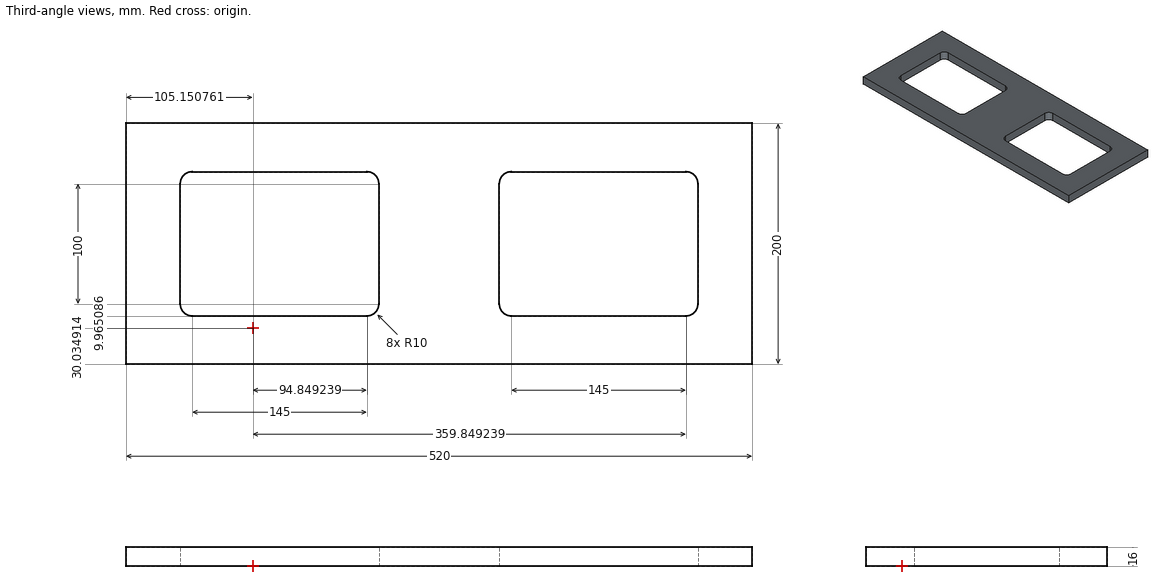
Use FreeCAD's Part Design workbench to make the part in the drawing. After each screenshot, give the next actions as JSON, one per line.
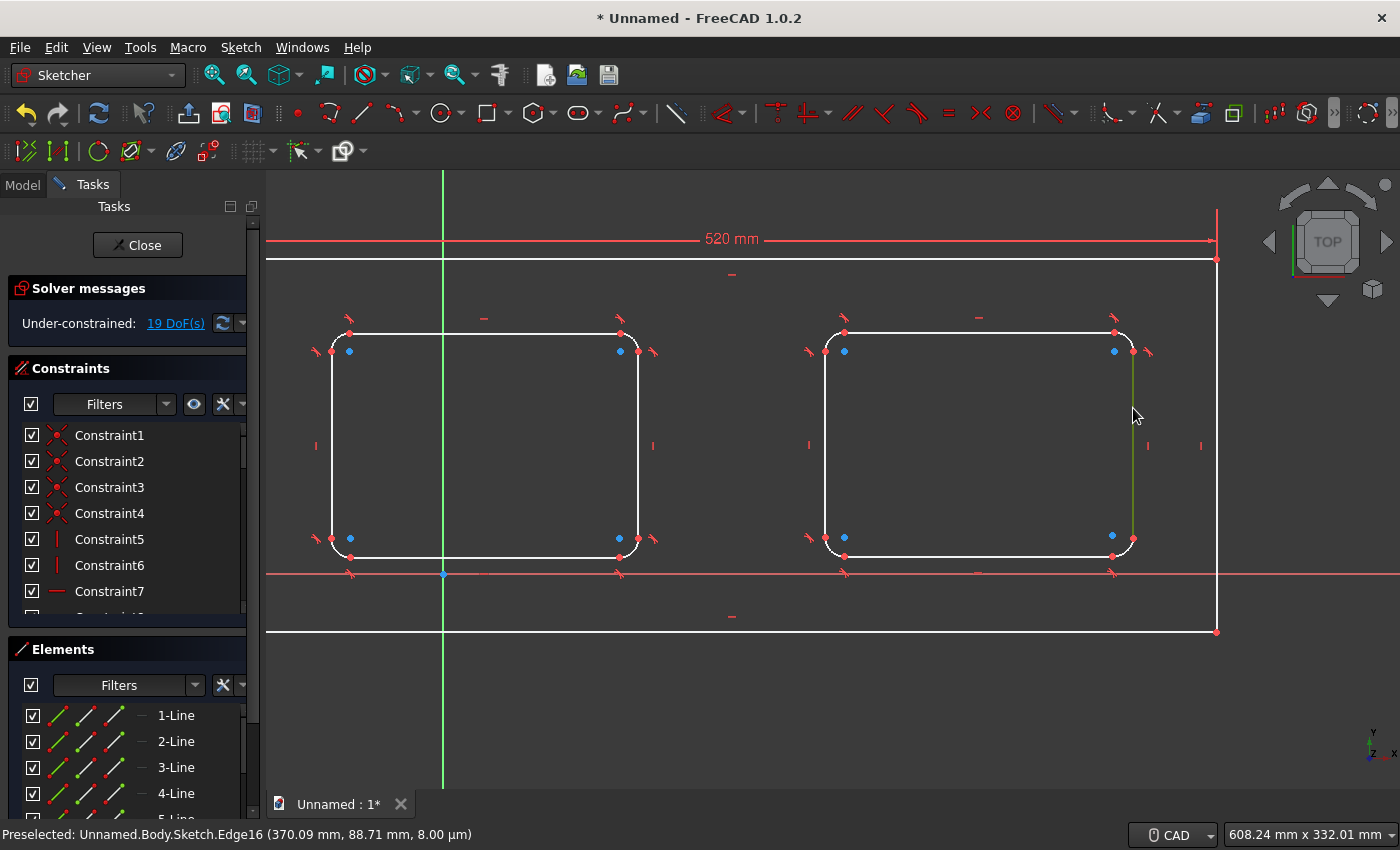
{"action": "left_click", "coordinate": [1127, 551]}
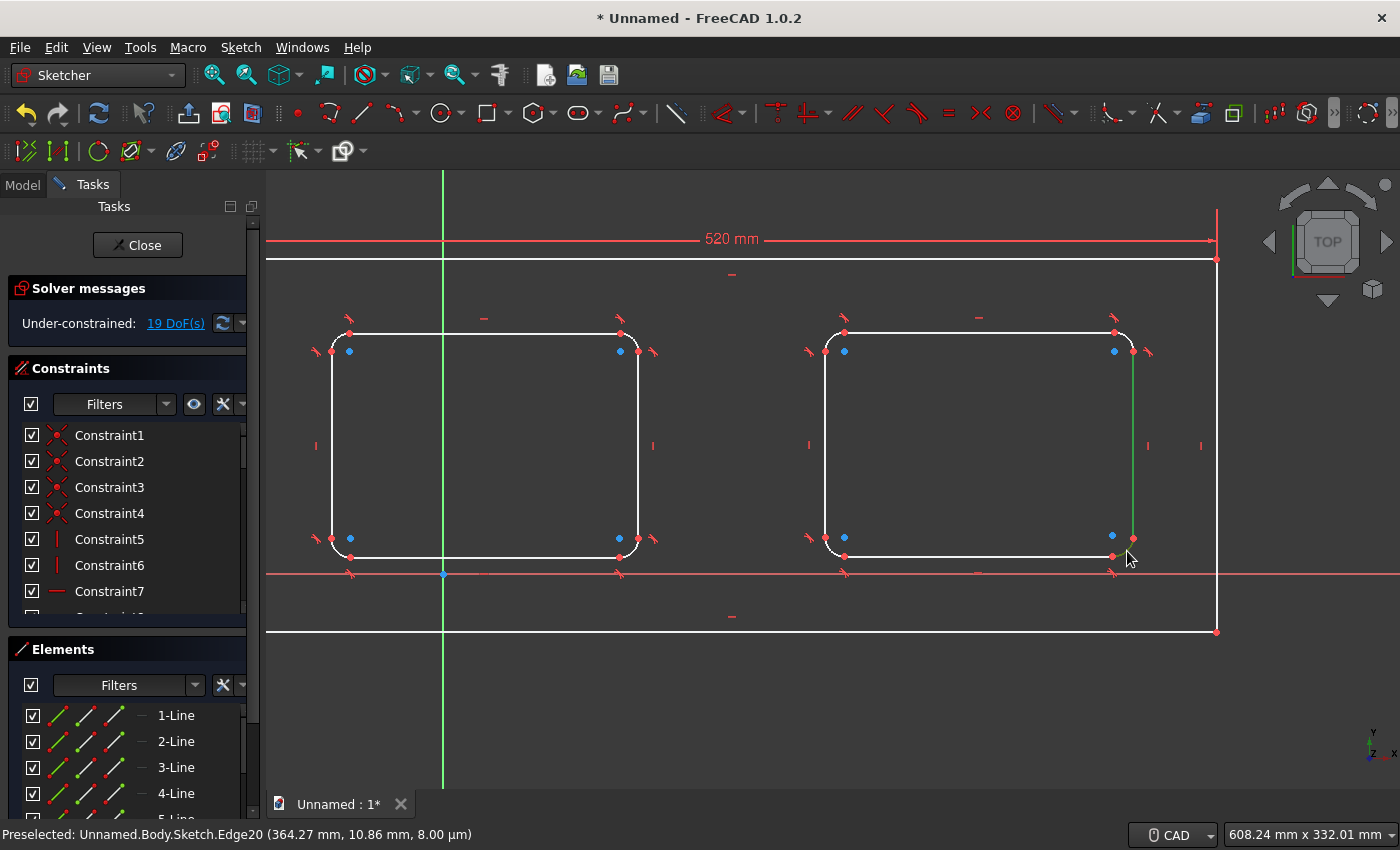
{"action": "key", "text": "t"}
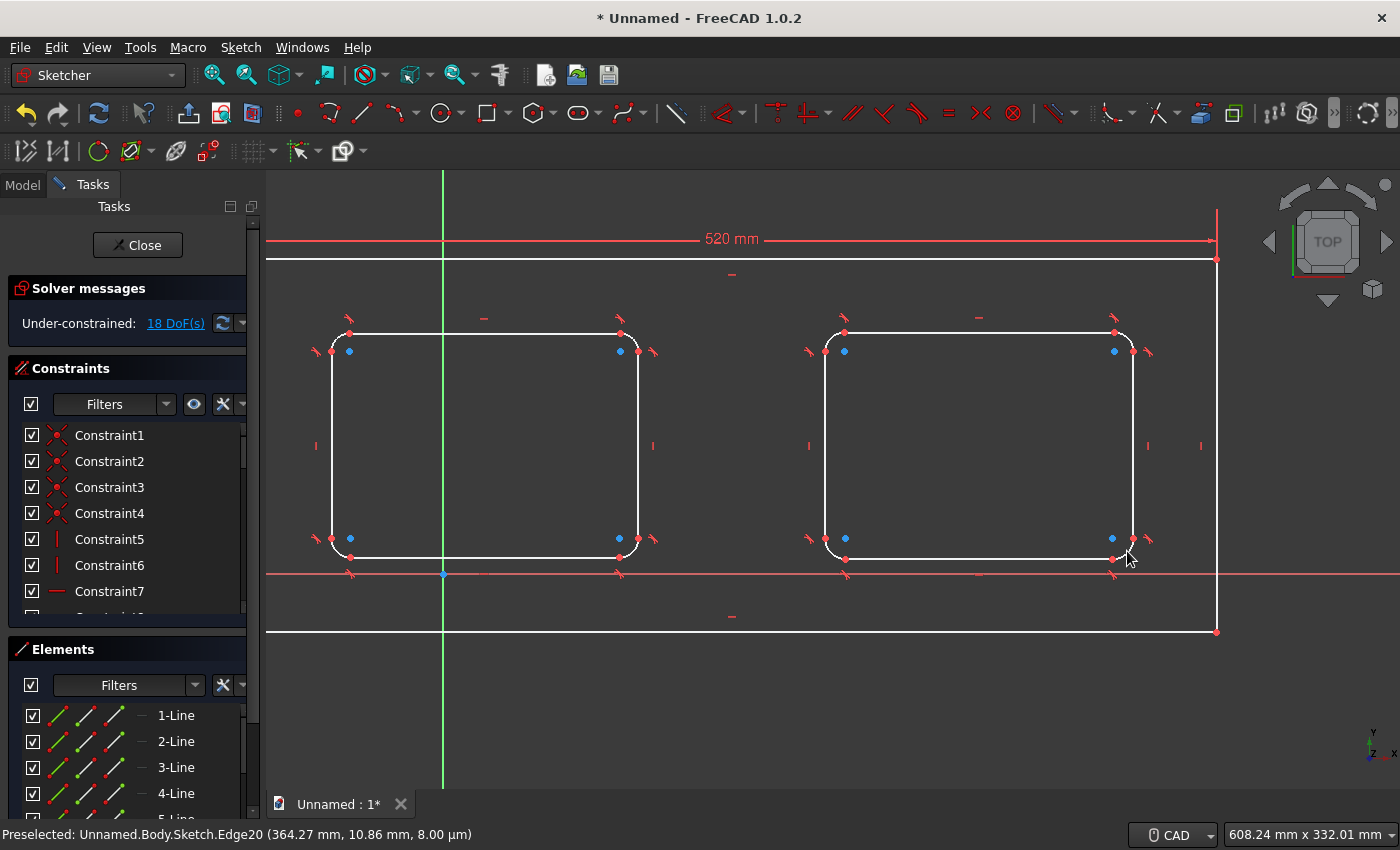
{"action": "scroll", "coordinate": [628, 556], "scroll_direction": "up", "scroll_amount": 3}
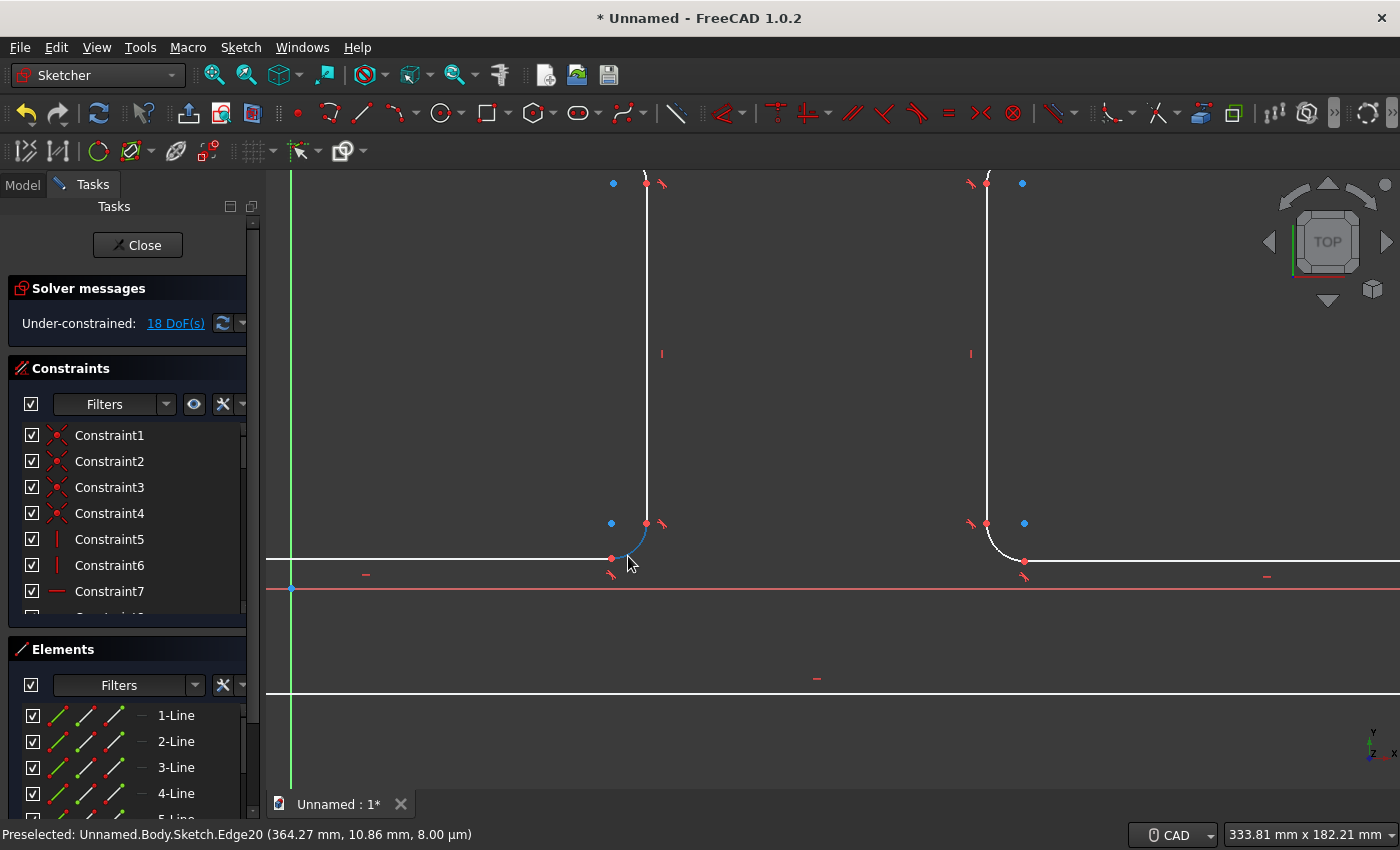
{"action": "left_click", "coordinate": [627, 555]}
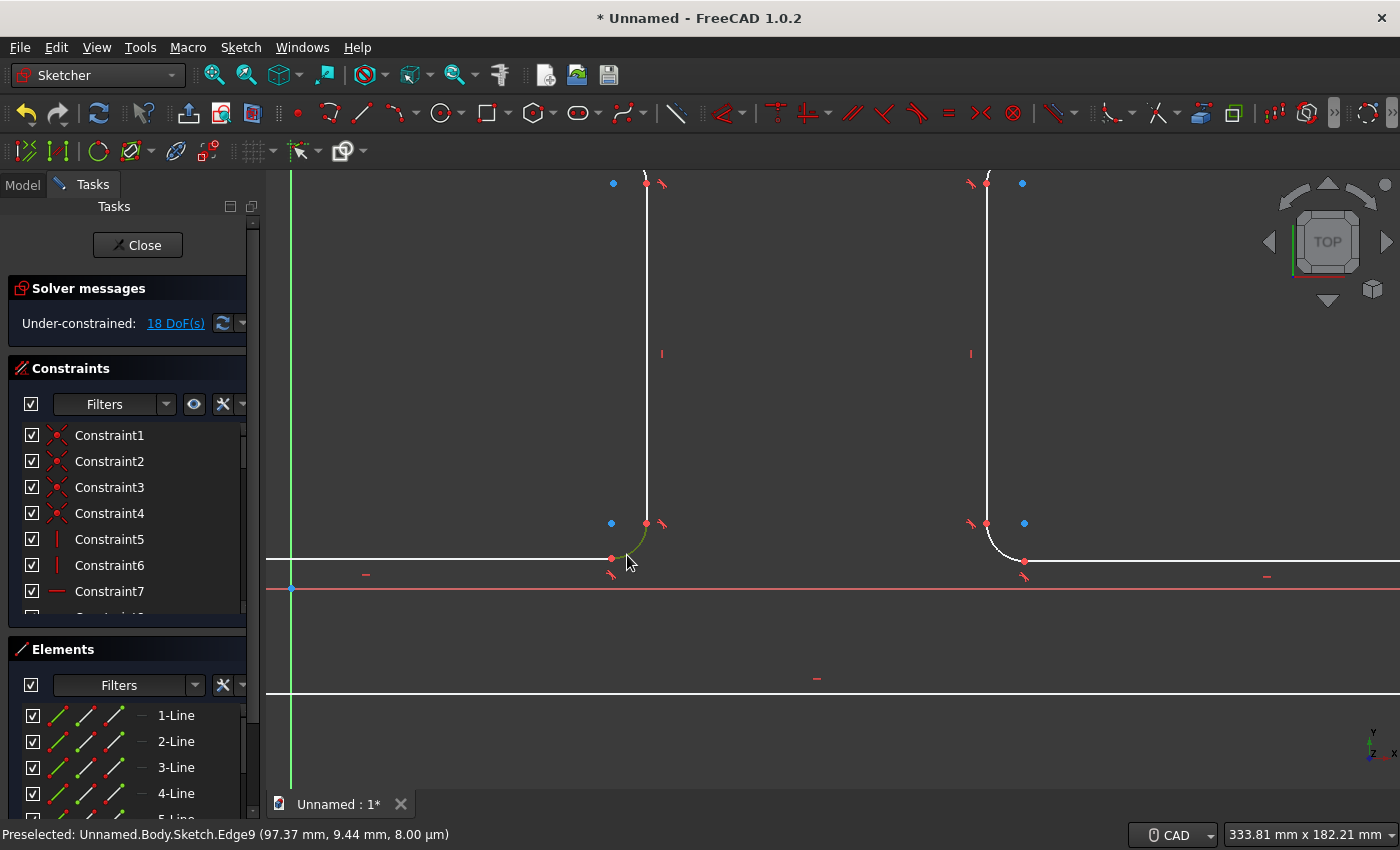
{"action": "scroll", "coordinate": [734, 554], "scroll_direction": "down", "scroll_amount": 5}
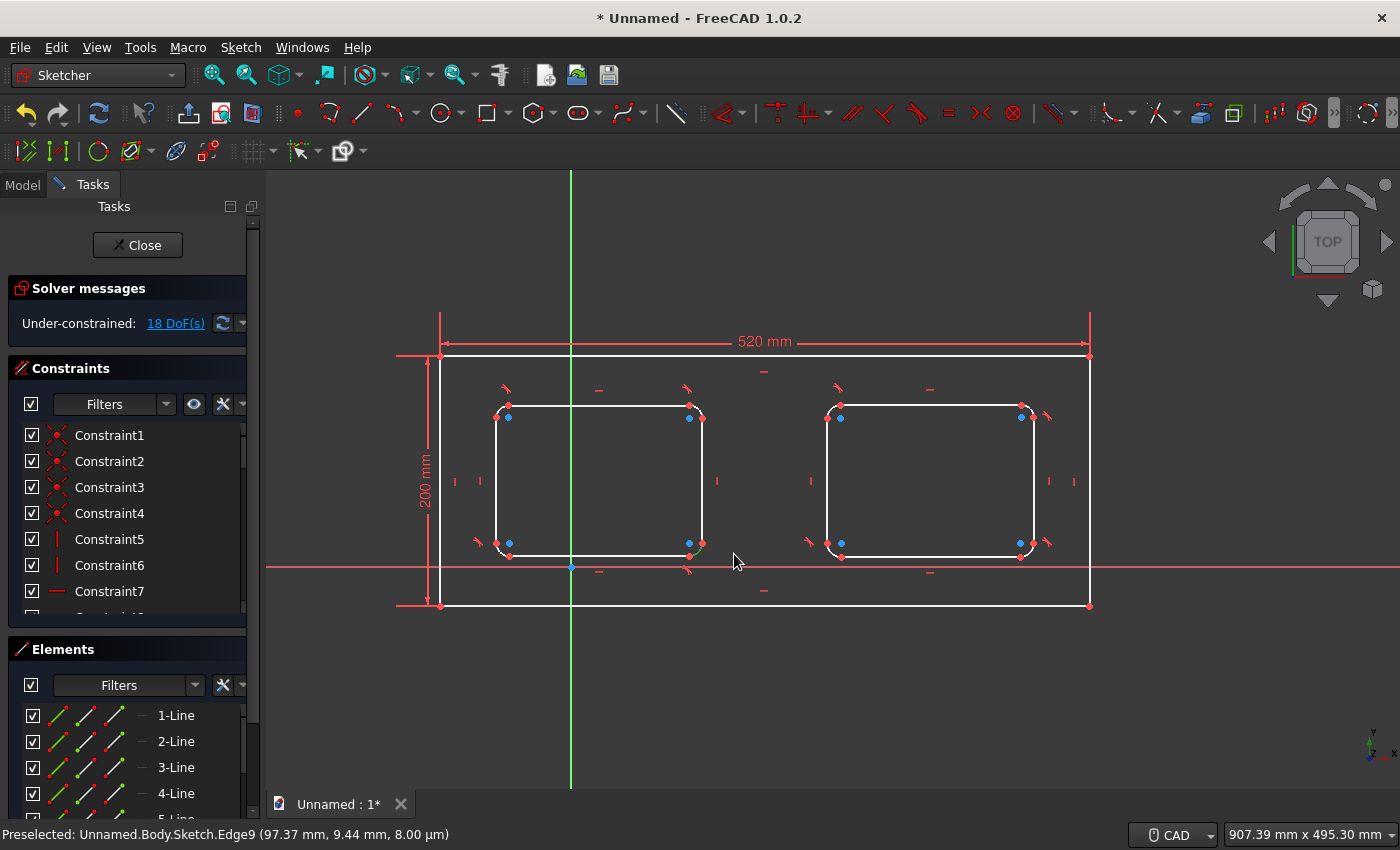
{"action": "scroll", "coordinate": [498, 549], "scroll_direction": "up", "scroll_amount": 5}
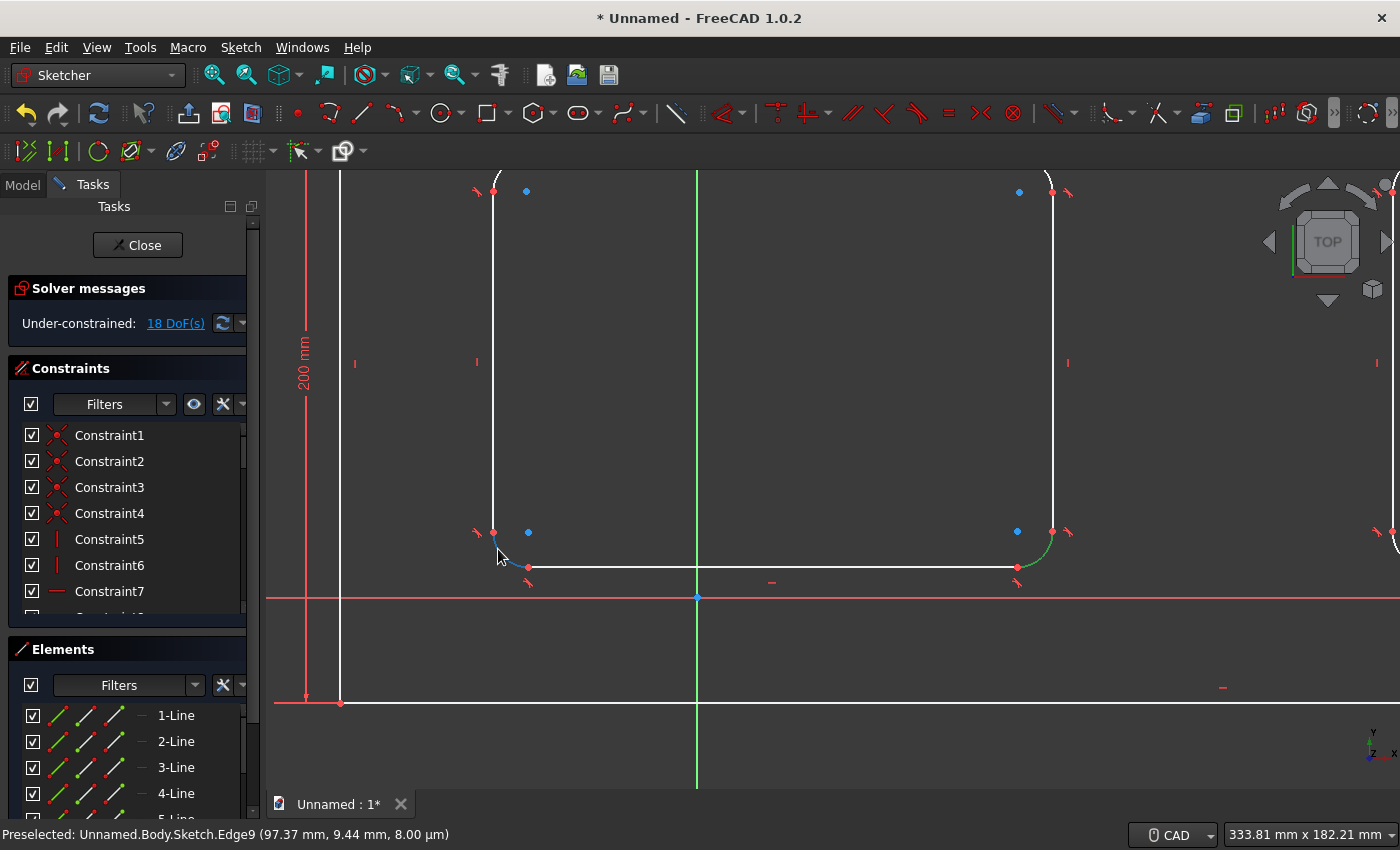
{"action": "left_click", "coordinate": [497, 548]}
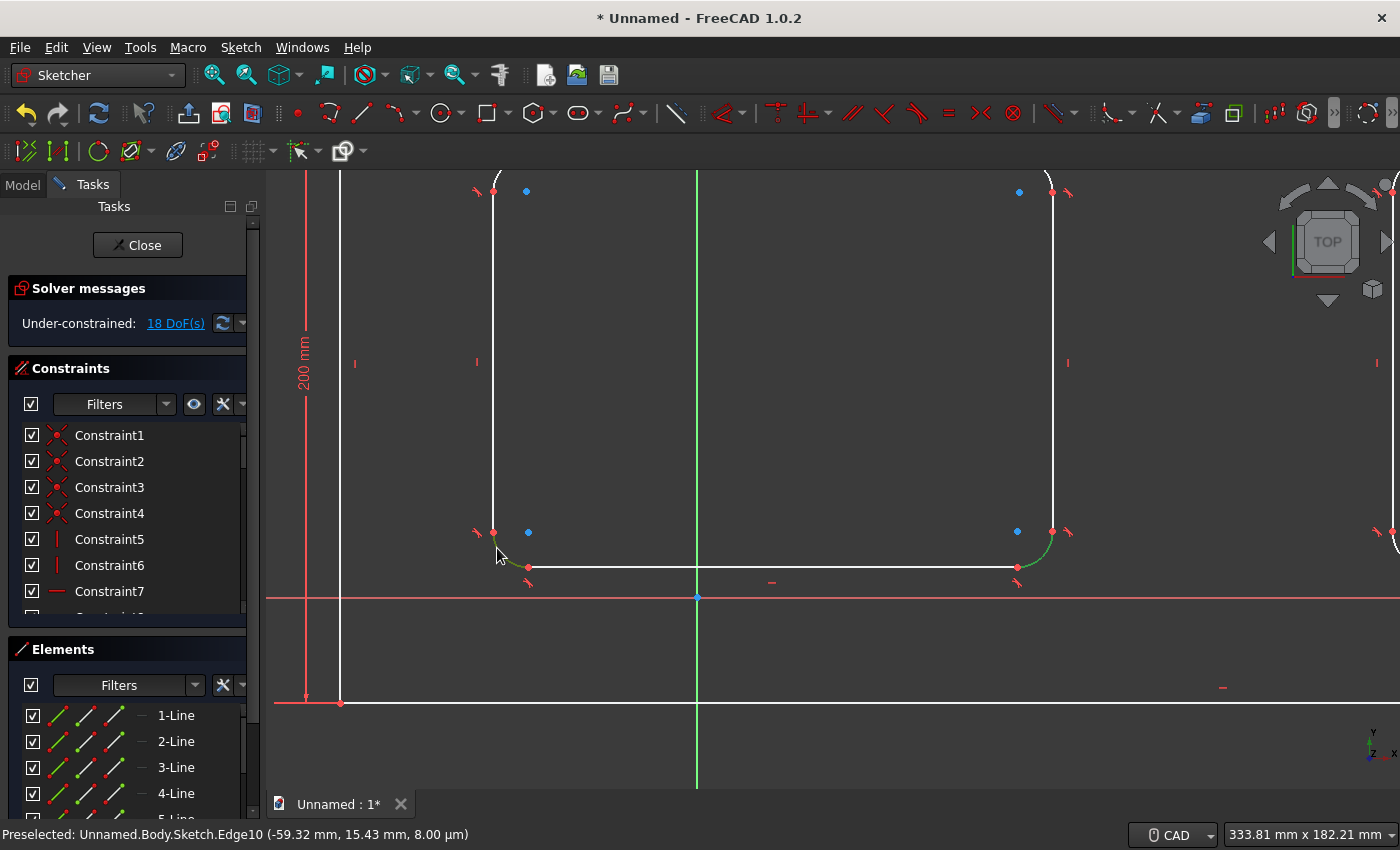
{"action": "scroll", "coordinate": [497, 549], "scroll_direction": "down", "scroll_amount": 5}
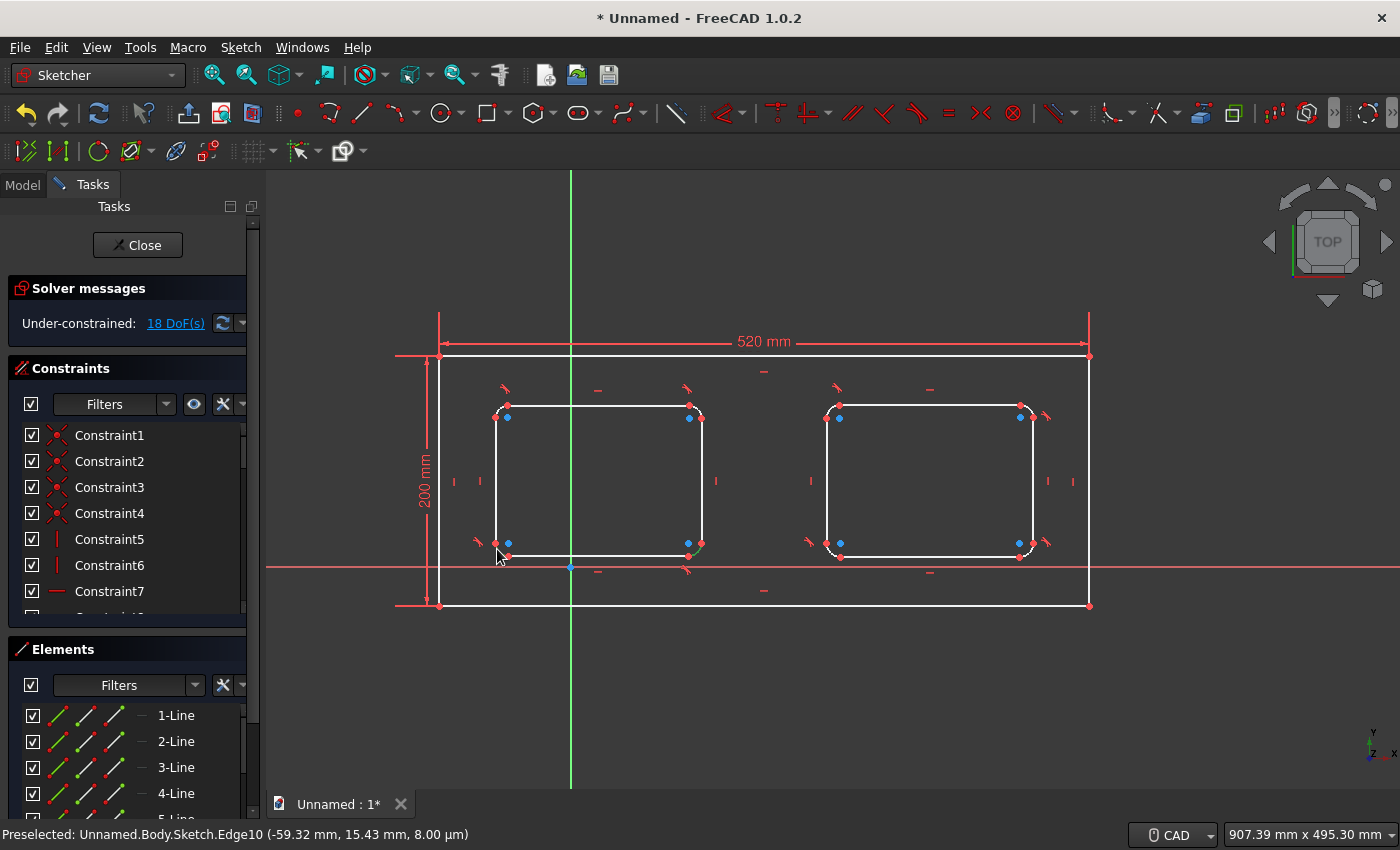
{"action": "scroll", "coordinate": [502, 407], "scroll_direction": "up", "scroll_amount": 5}